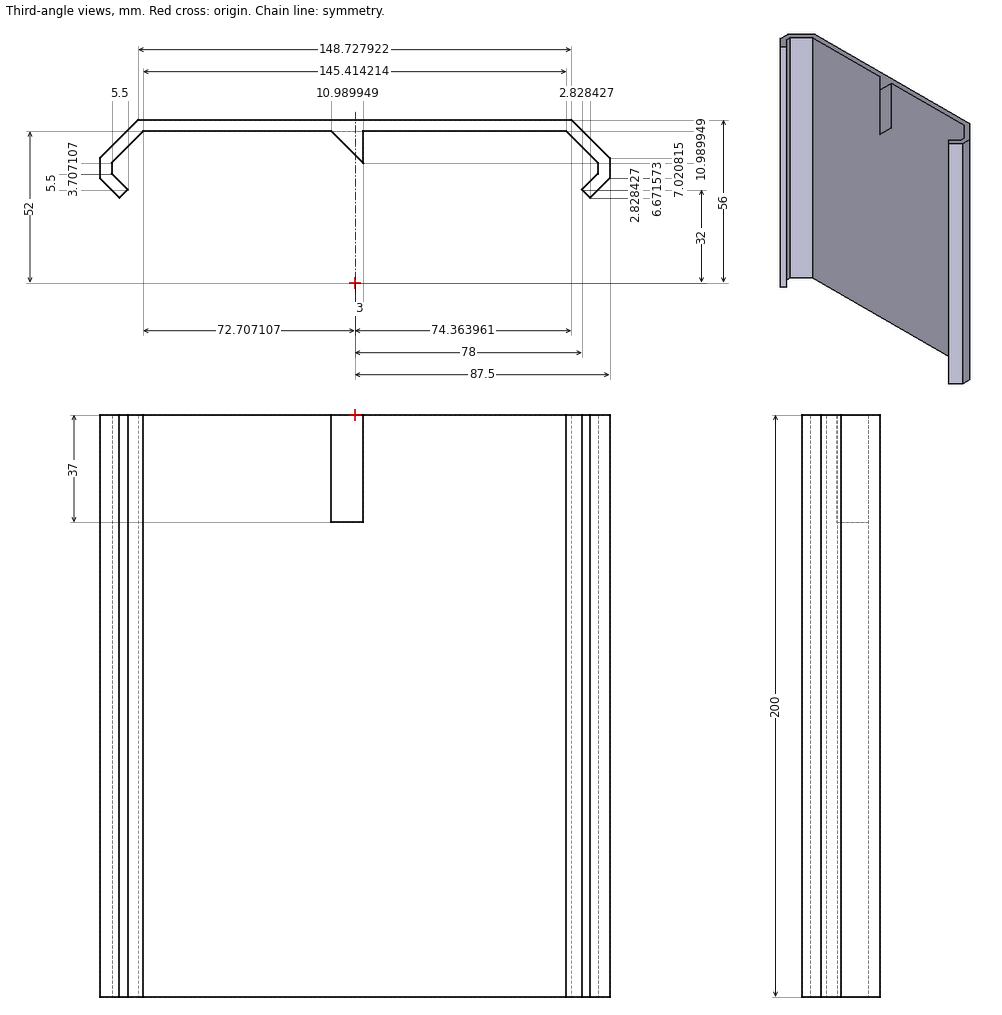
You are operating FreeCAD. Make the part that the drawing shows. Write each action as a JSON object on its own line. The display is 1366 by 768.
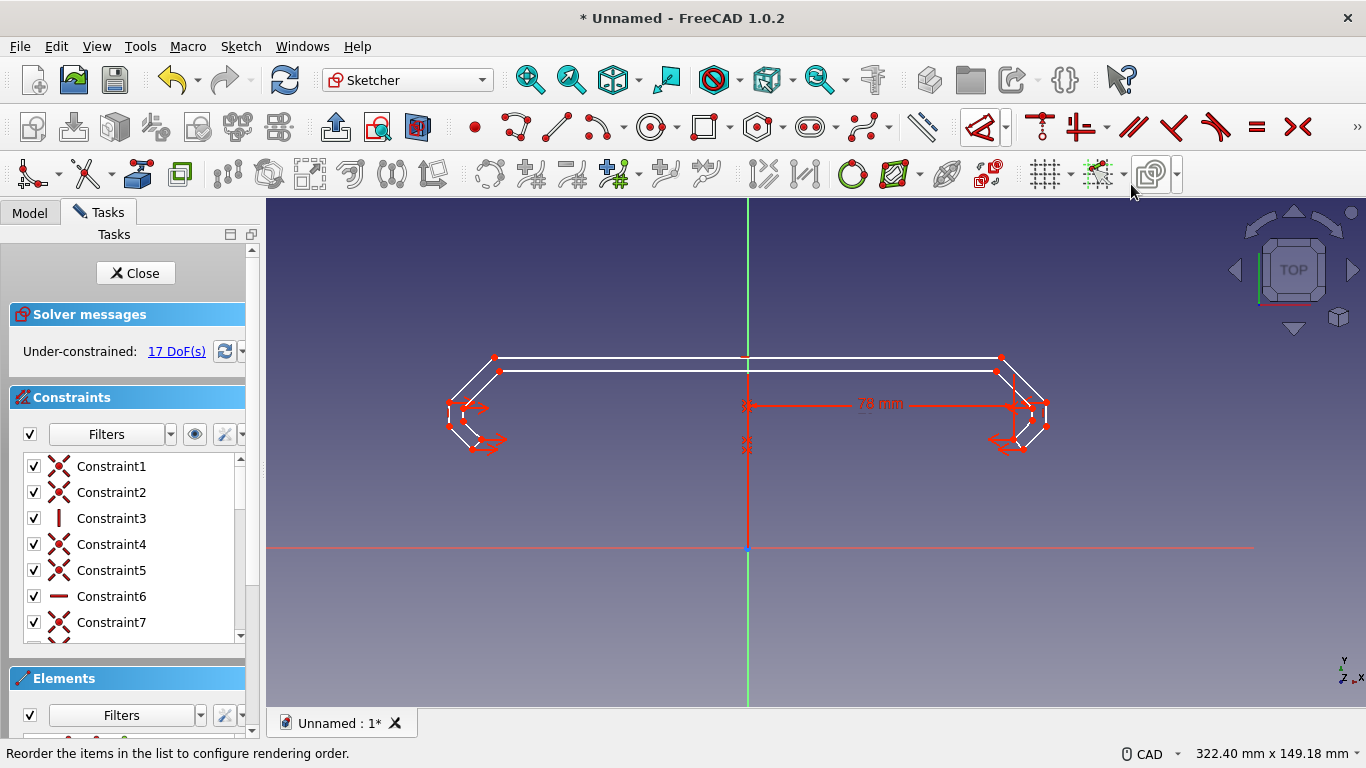
{"action": "left_click", "coordinate": [1014, 440]}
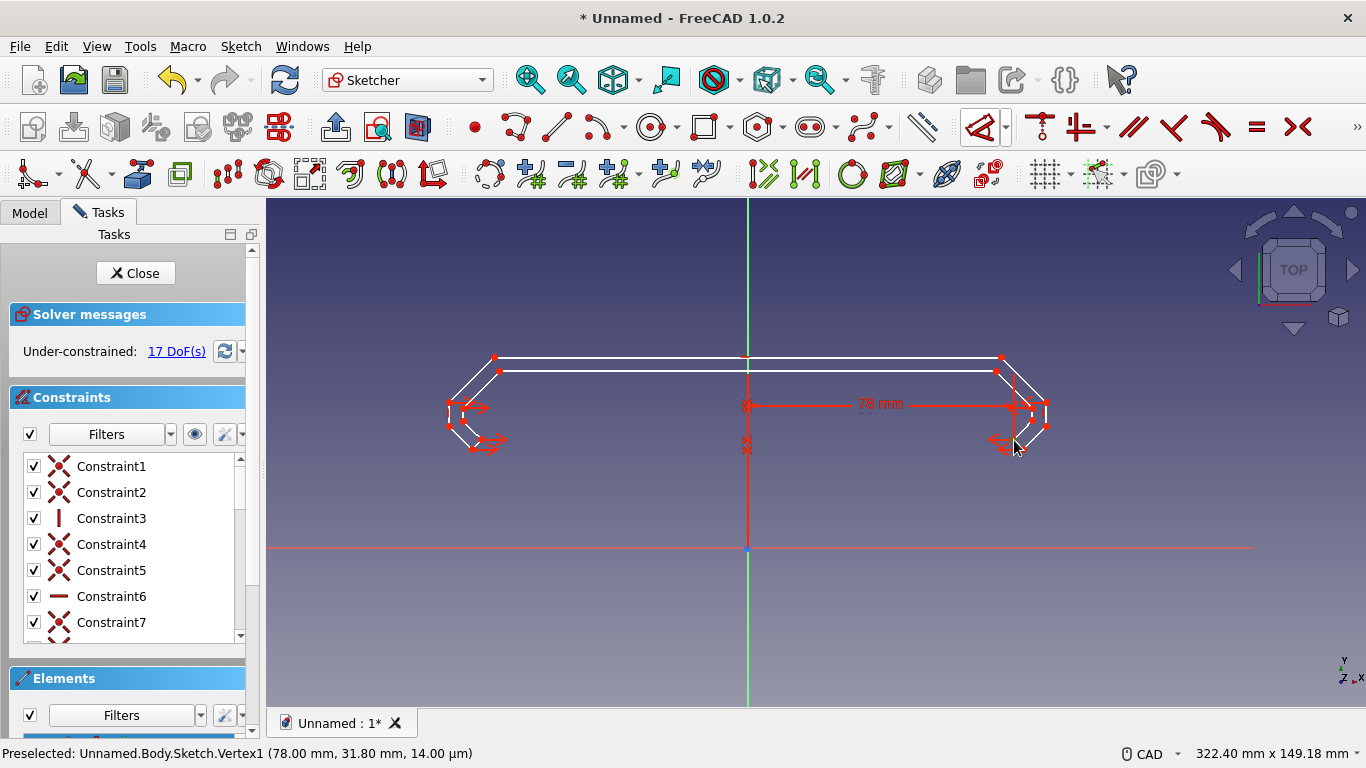
{"action": "left_click", "coordinate": [1006, 128]}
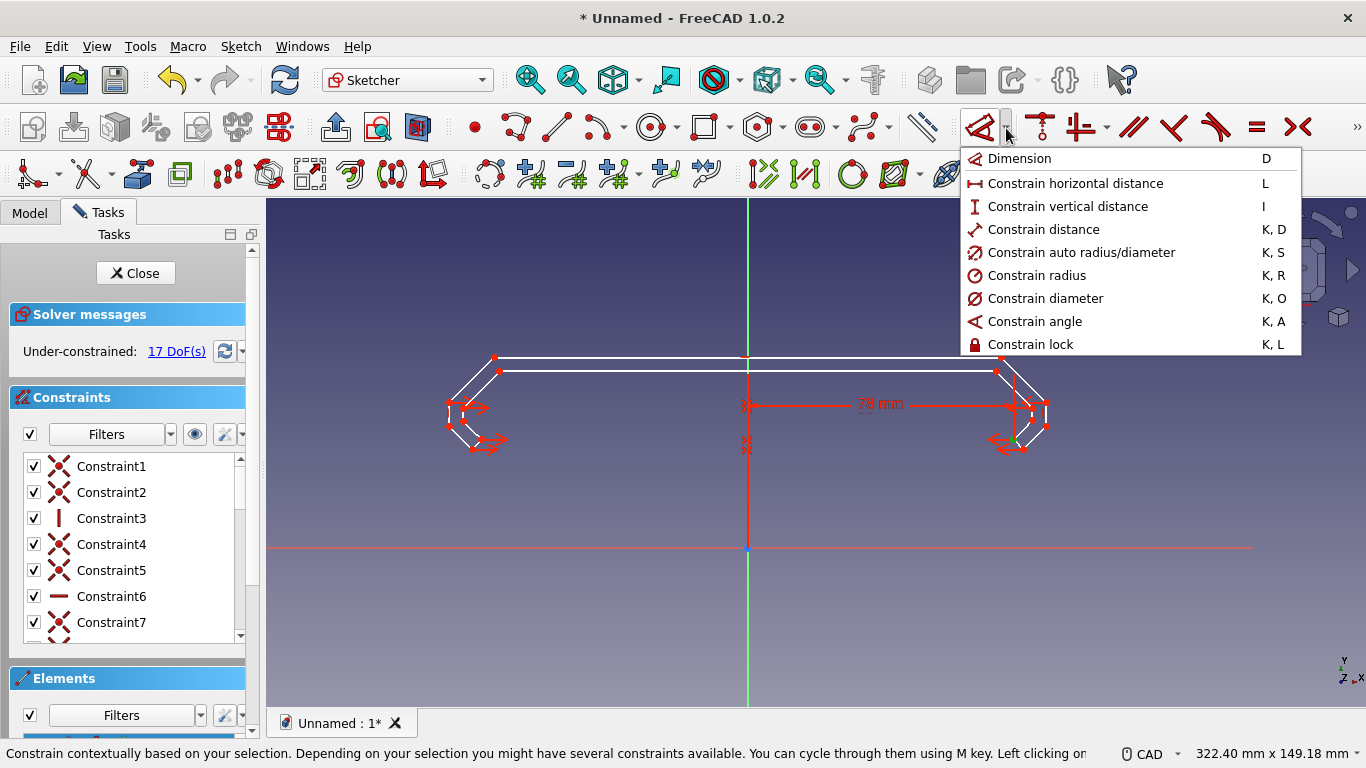
{"action": "left_click", "coordinate": [1131, 206]}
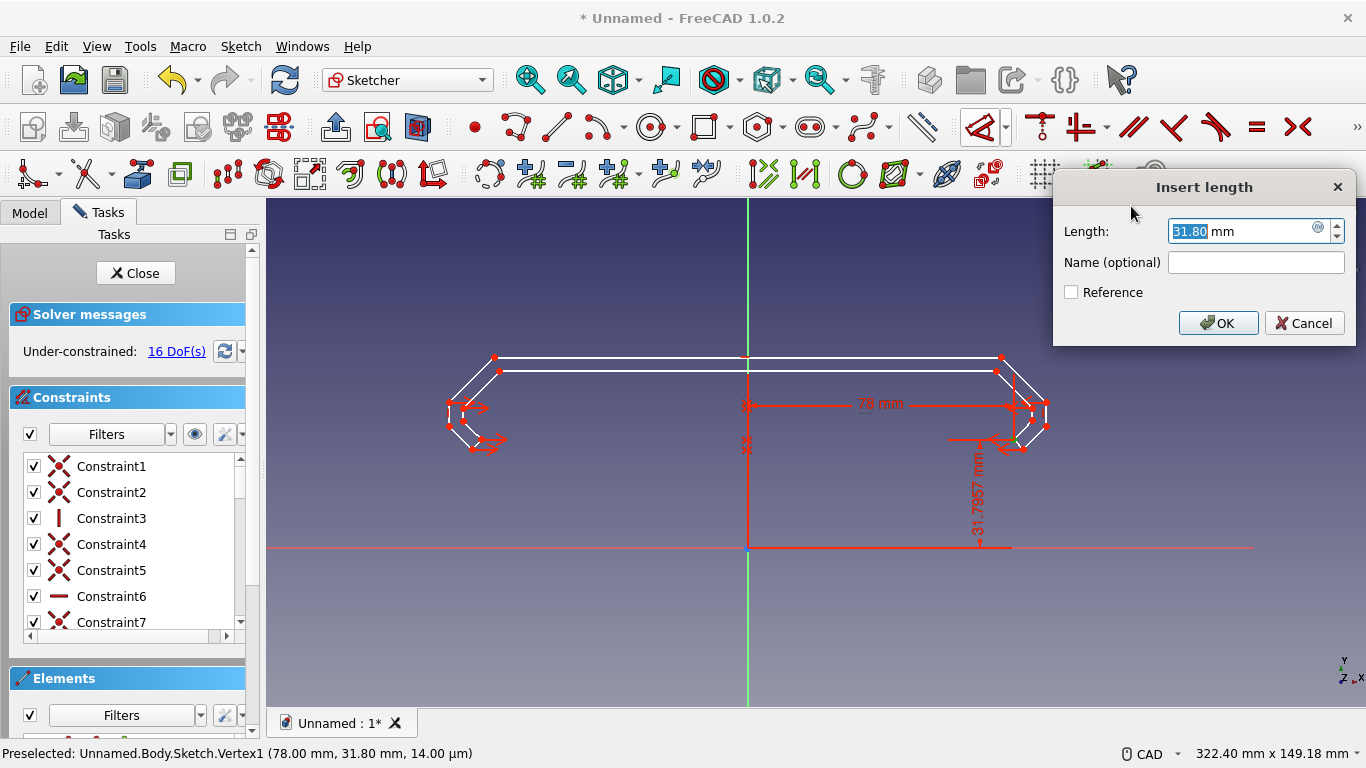
{"action": "type", "text": "32"}
{"action": "key", "text": "Return"}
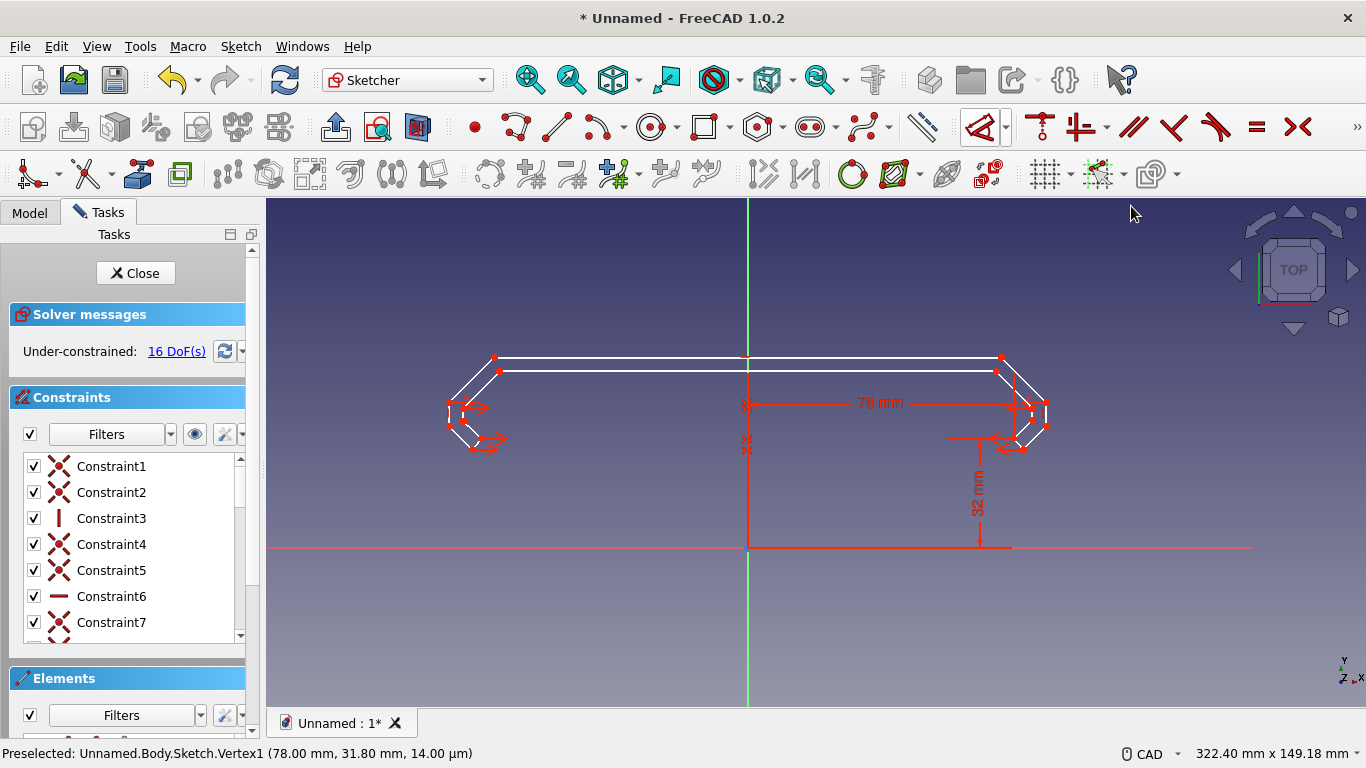
{"action": "left_click", "coordinate": [1001, 358]}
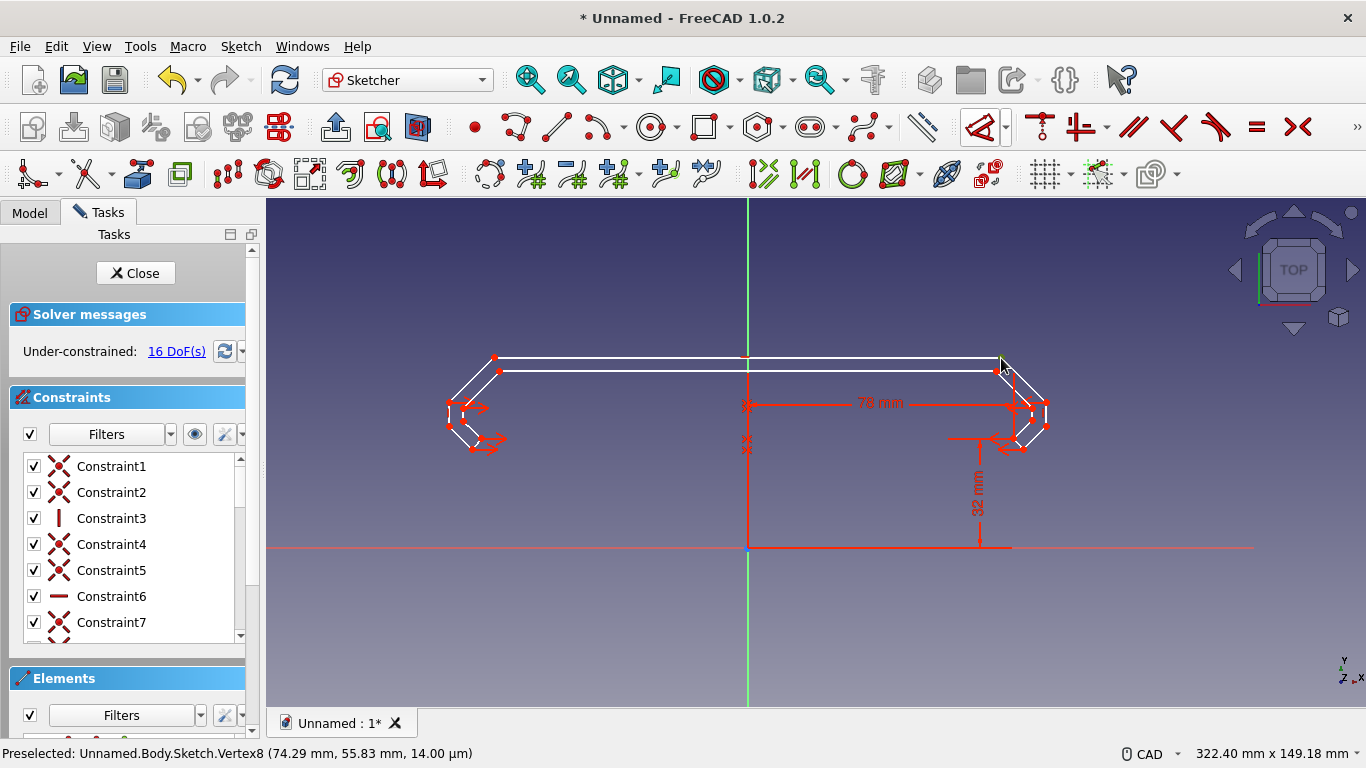
{"action": "left_click", "coordinate": [1006, 128]}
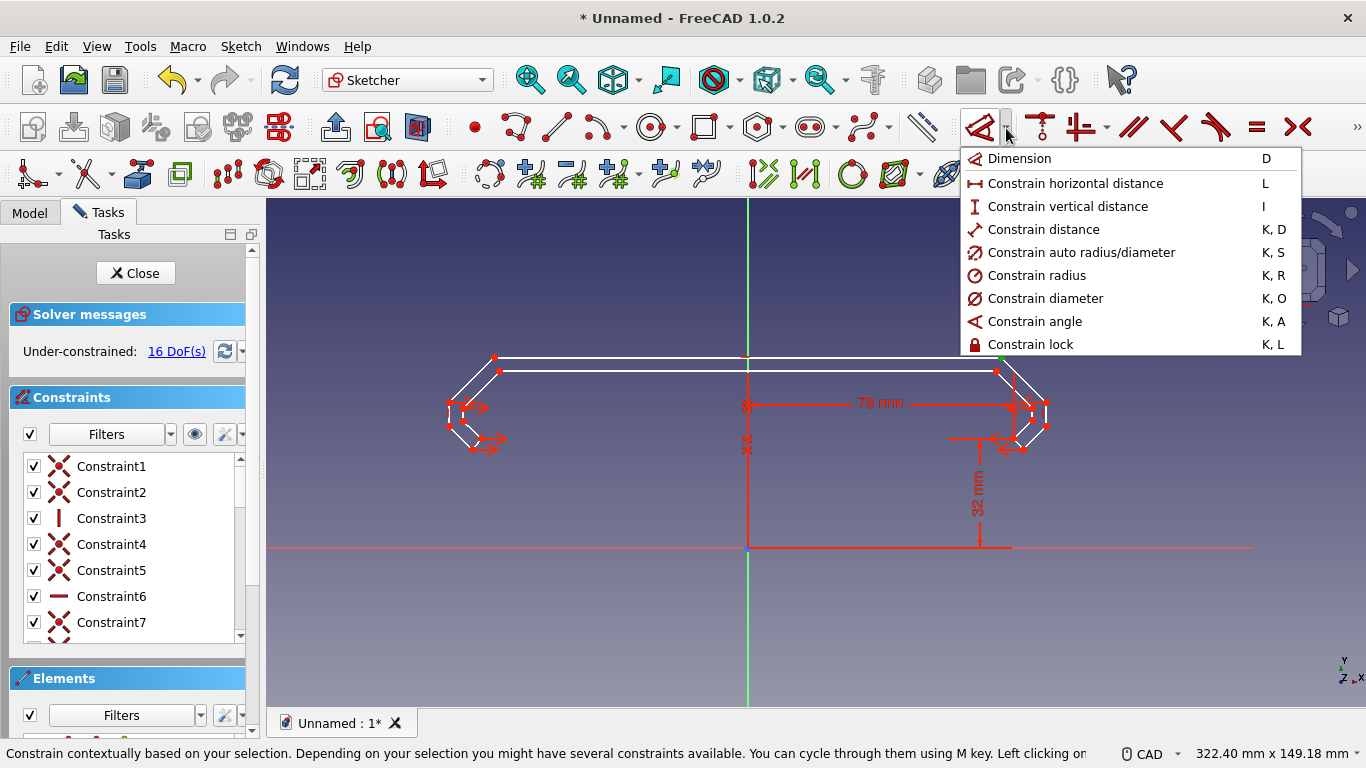
{"action": "left_click", "coordinate": [1131, 206]}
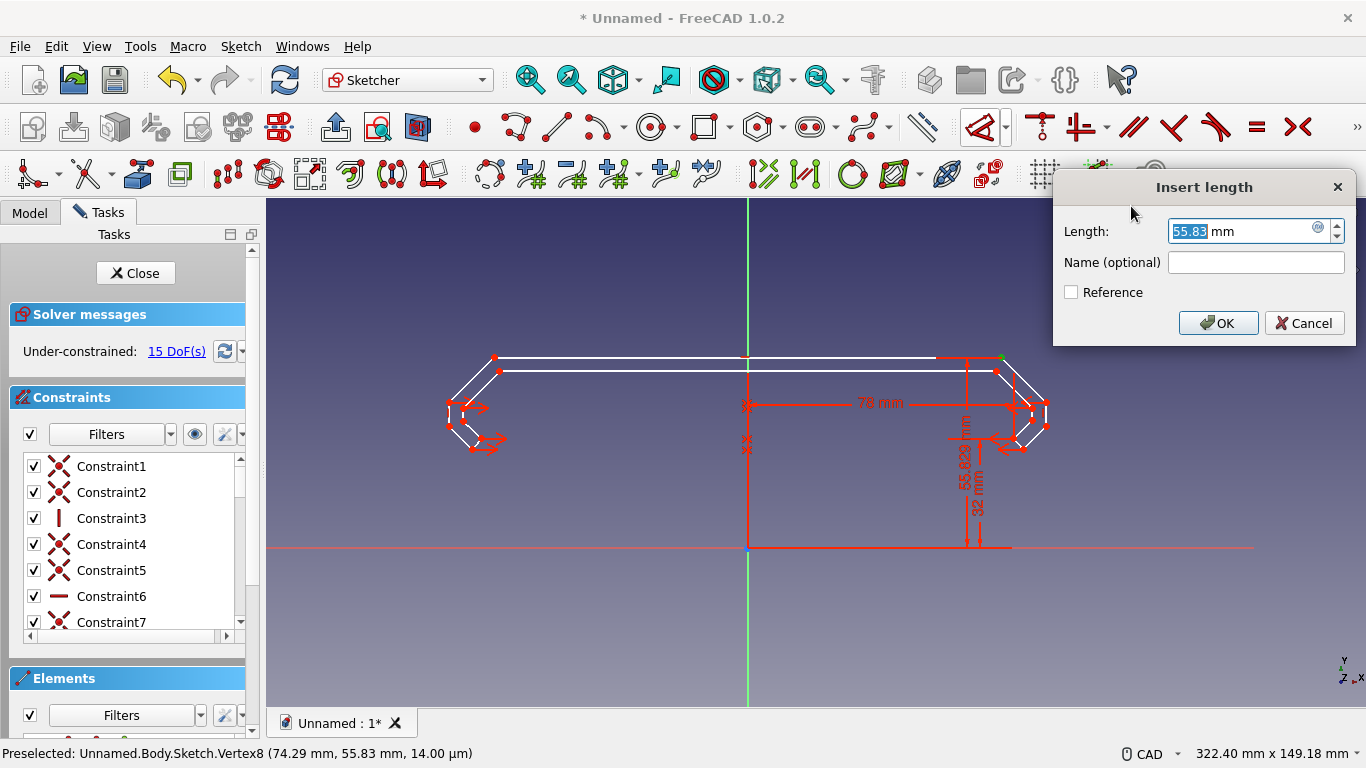
{"action": "type", "text": "56"}
{"action": "key", "text": "Return"}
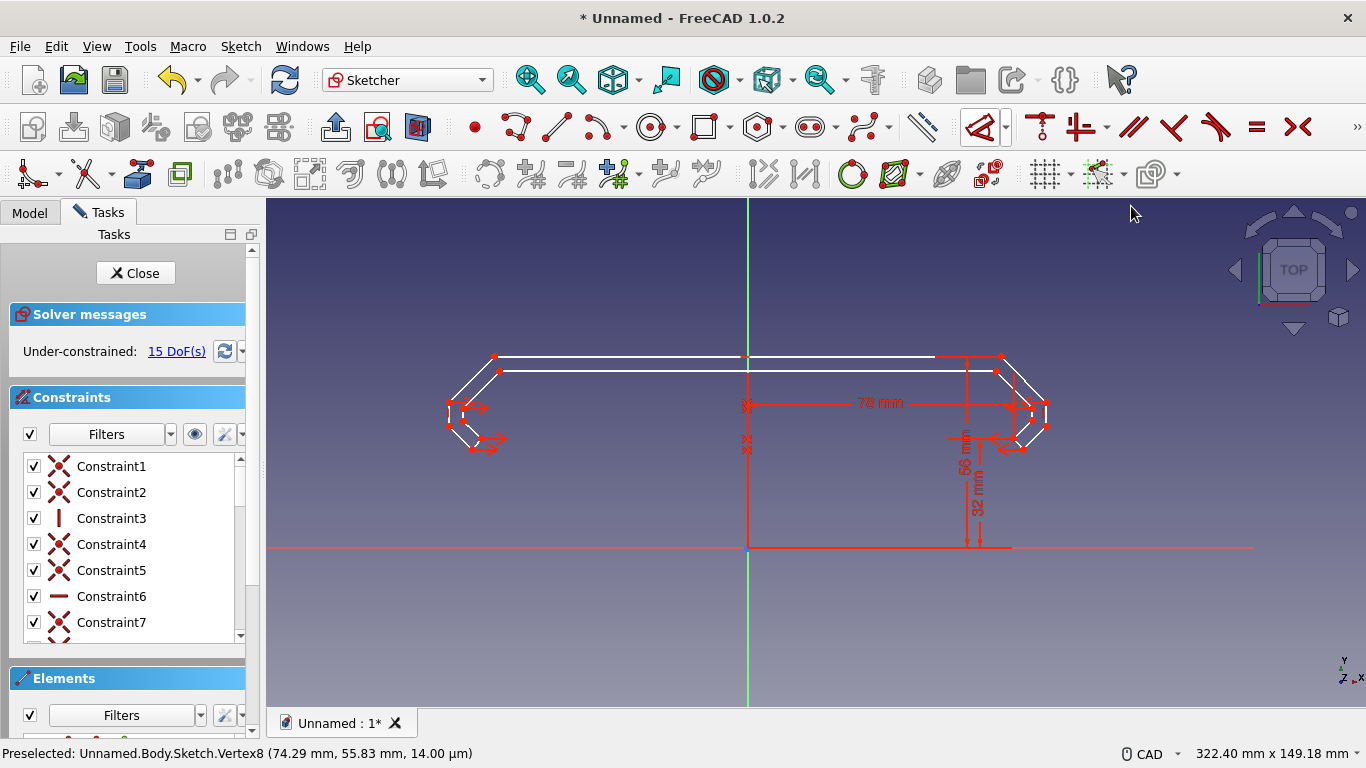
{"action": "left_click", "coordinate": [500, 371]}